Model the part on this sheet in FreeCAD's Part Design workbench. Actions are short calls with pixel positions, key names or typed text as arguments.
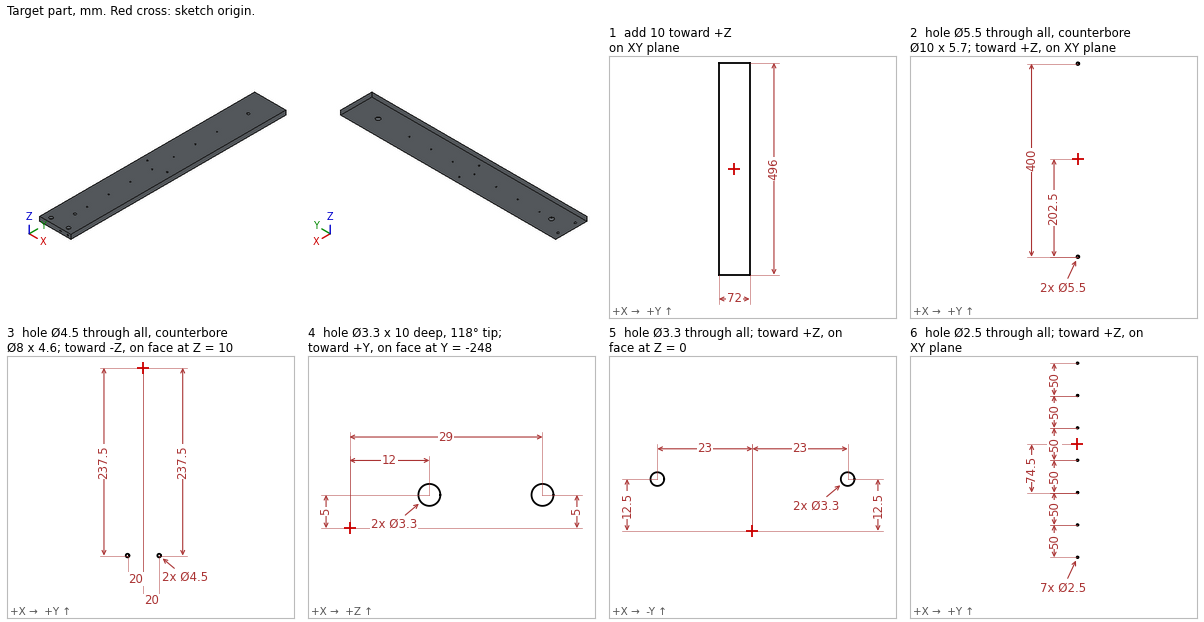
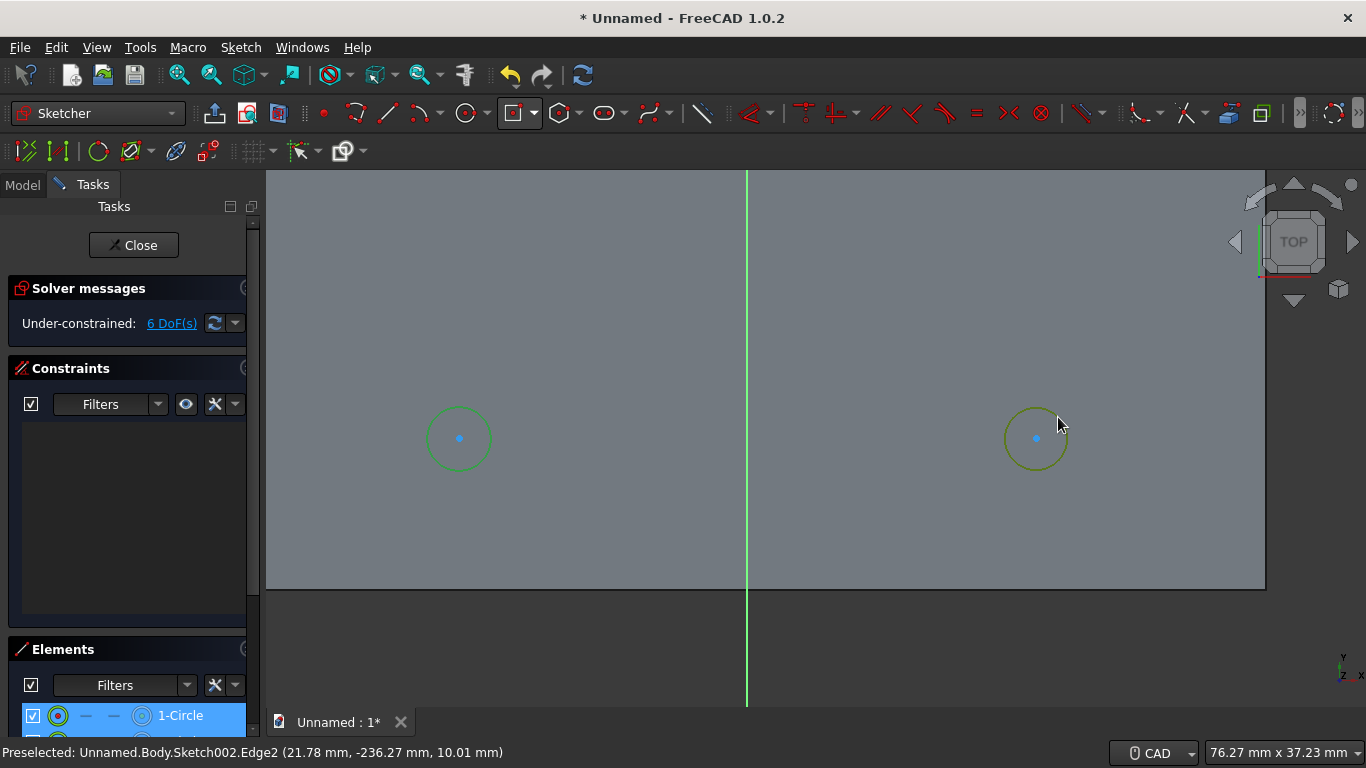
key(e)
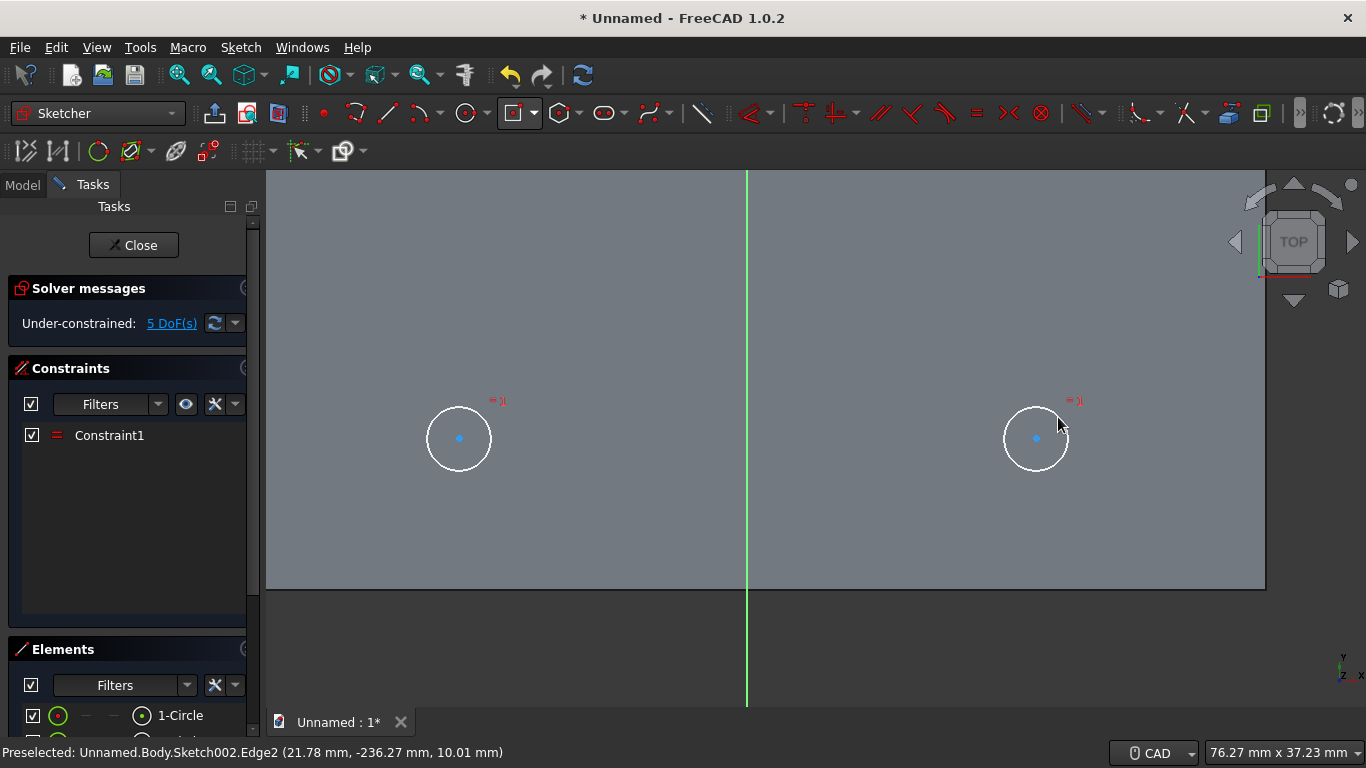
click(750, 114)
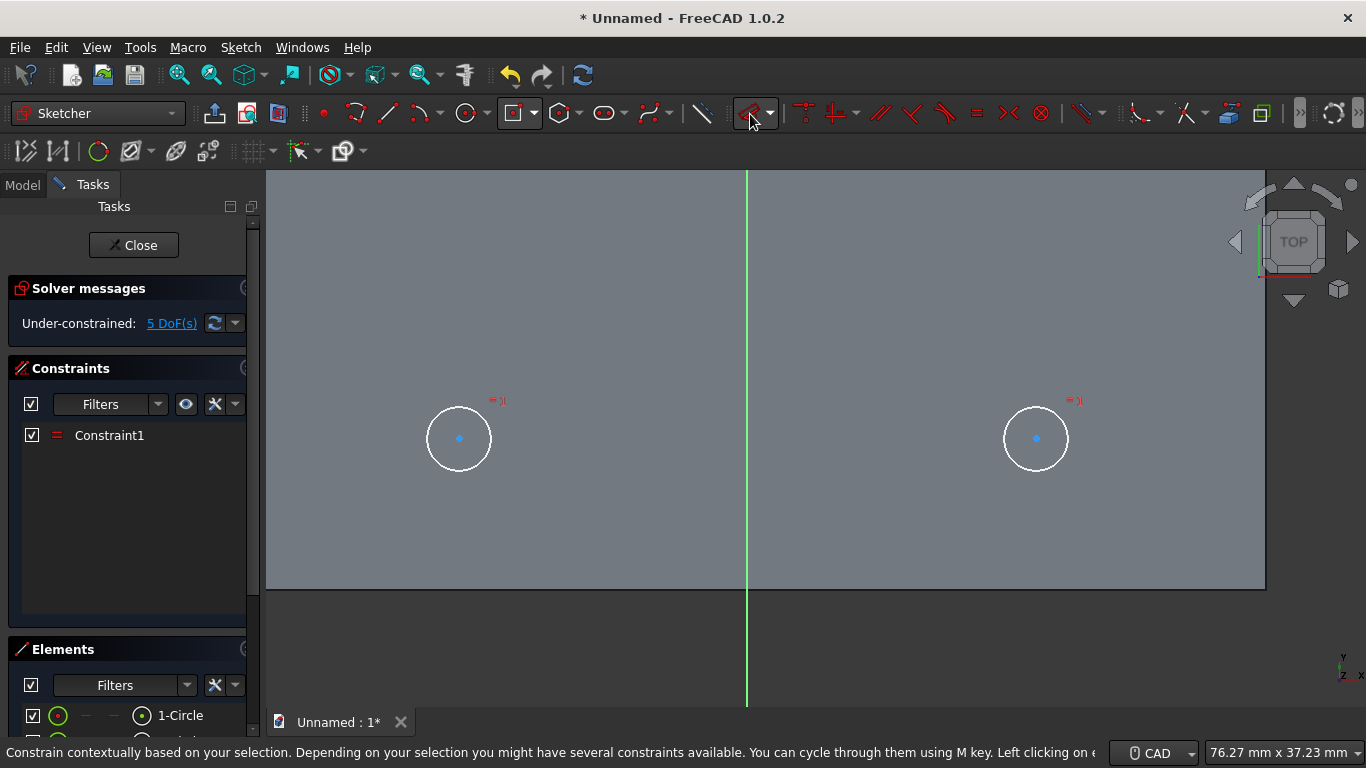
click(481, 416)
click(503, 393)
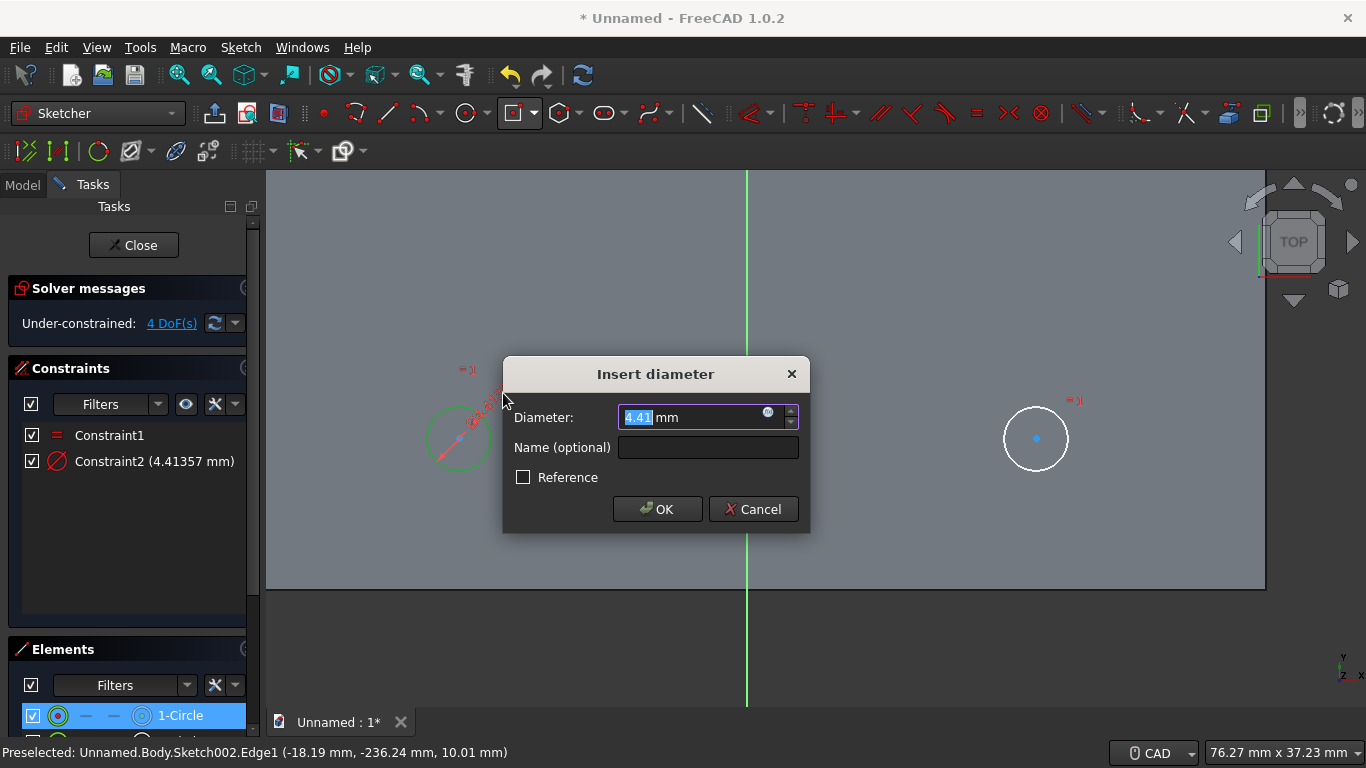
text(4.5)
key(Return)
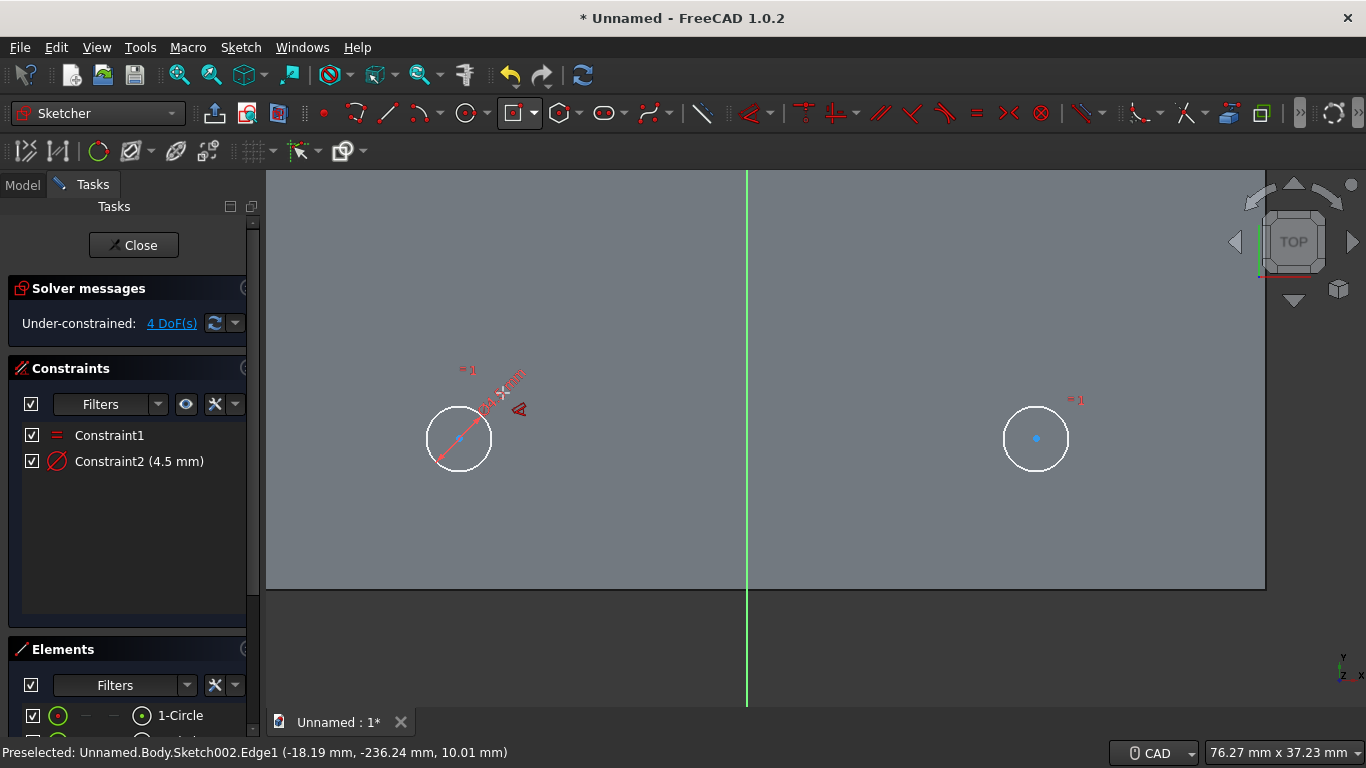
click(459, 439)
click(603, 473)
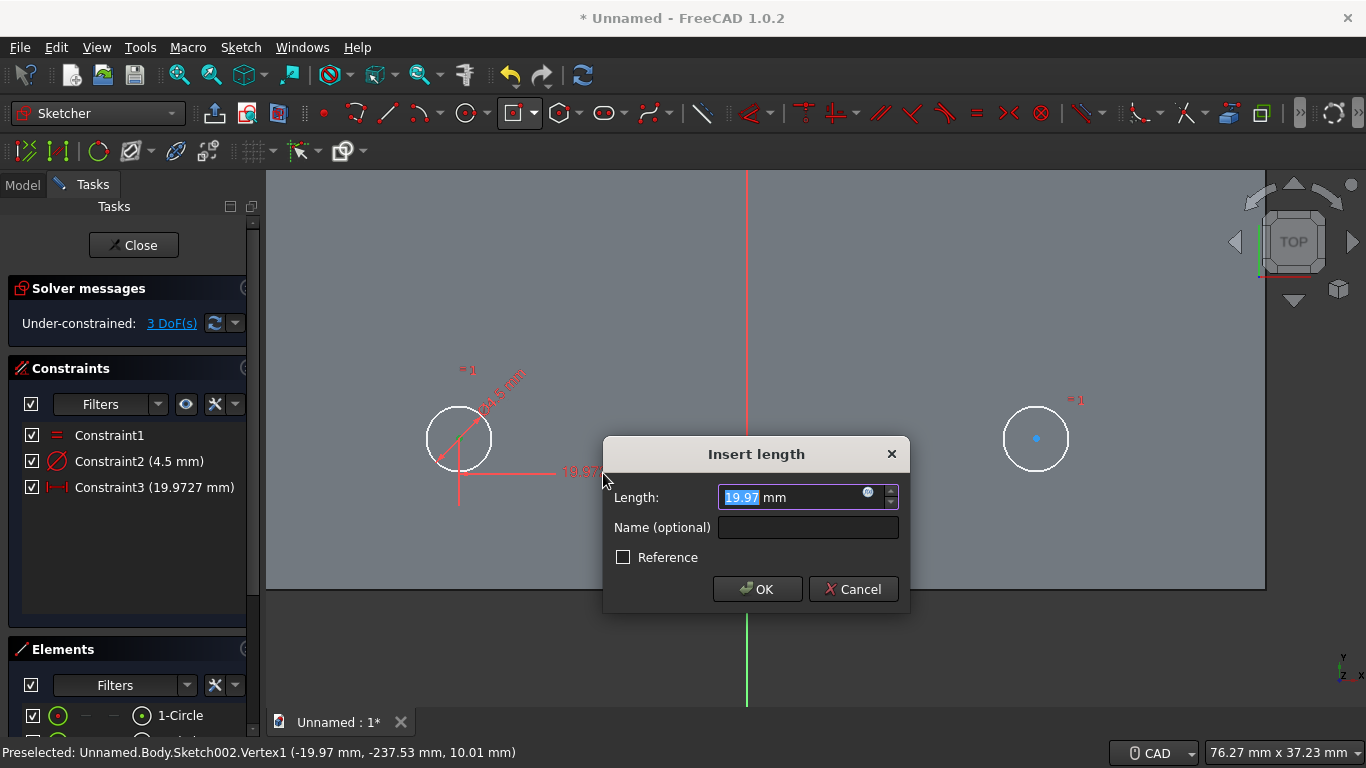
text(20)
key(Return)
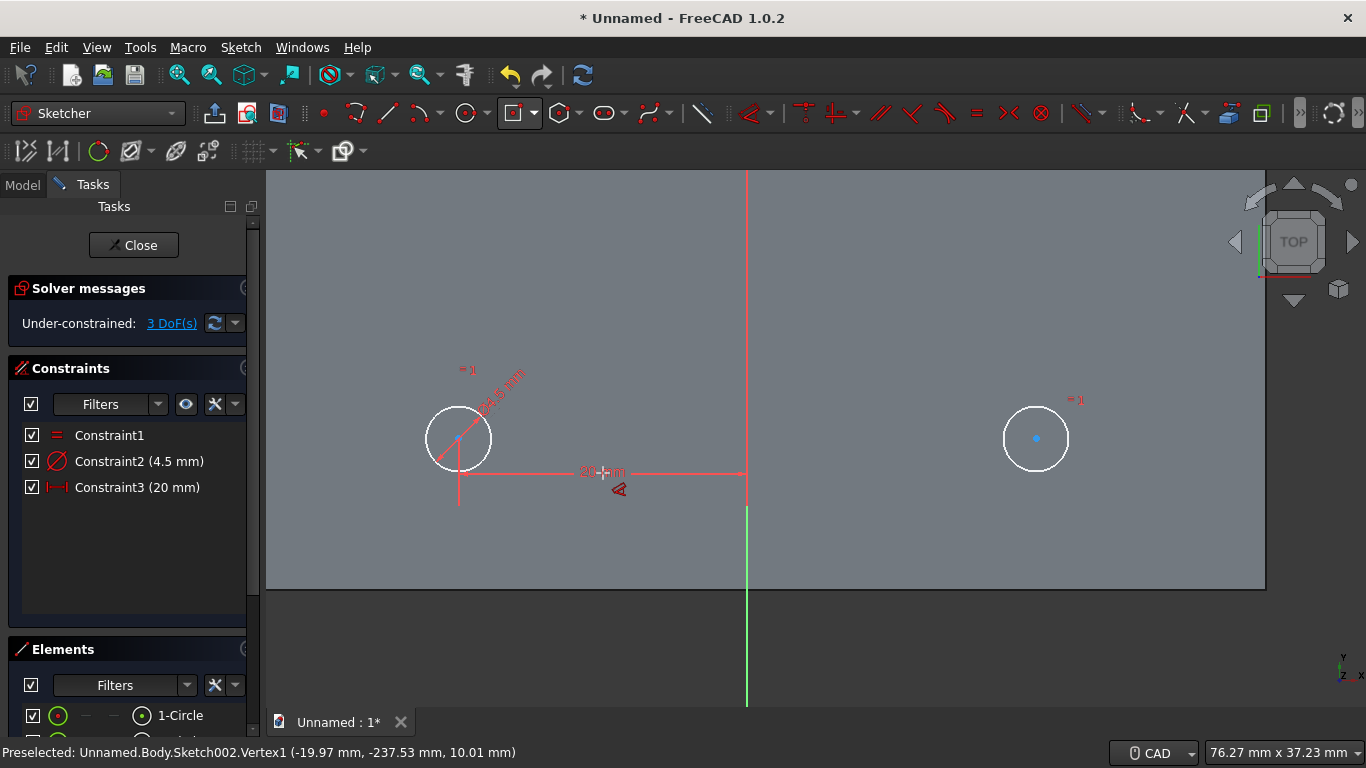
click(1036, 439)
click(892, 473)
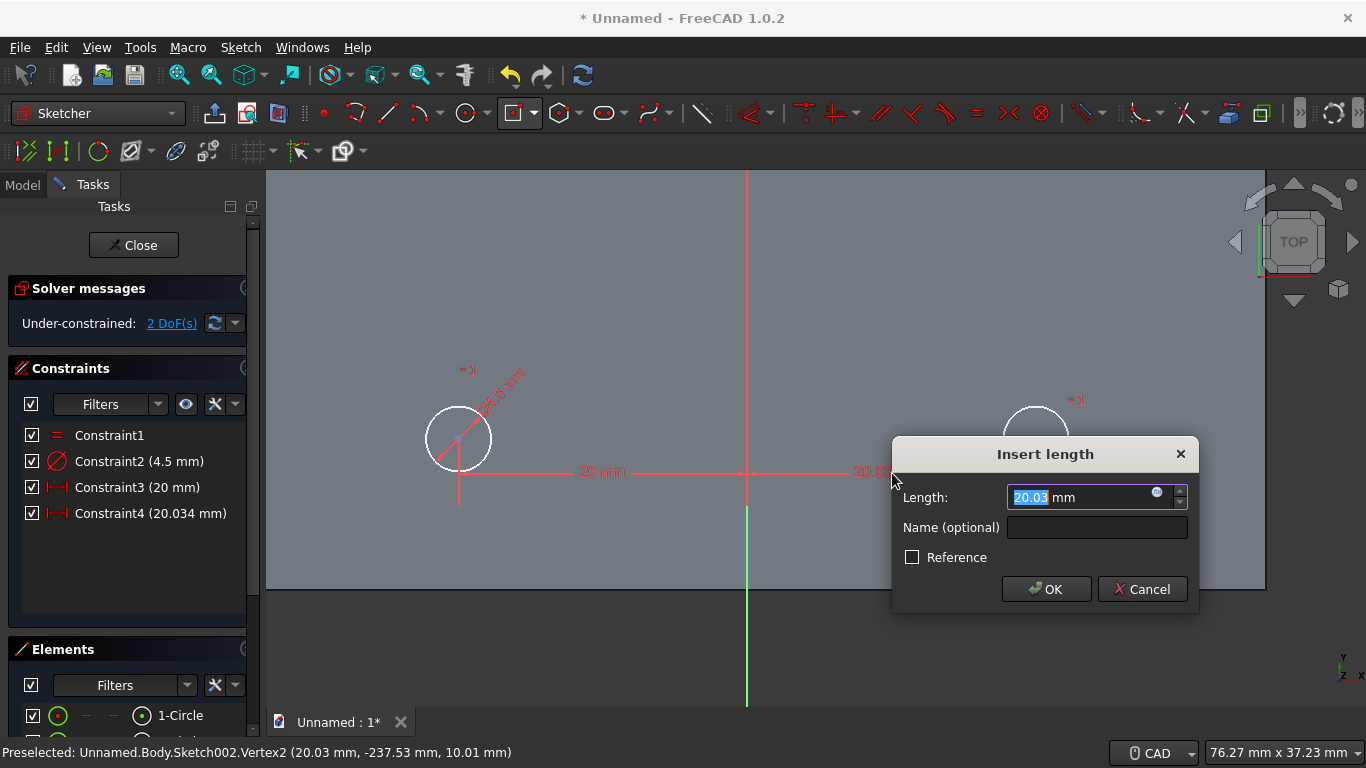
text(20)
key(Return)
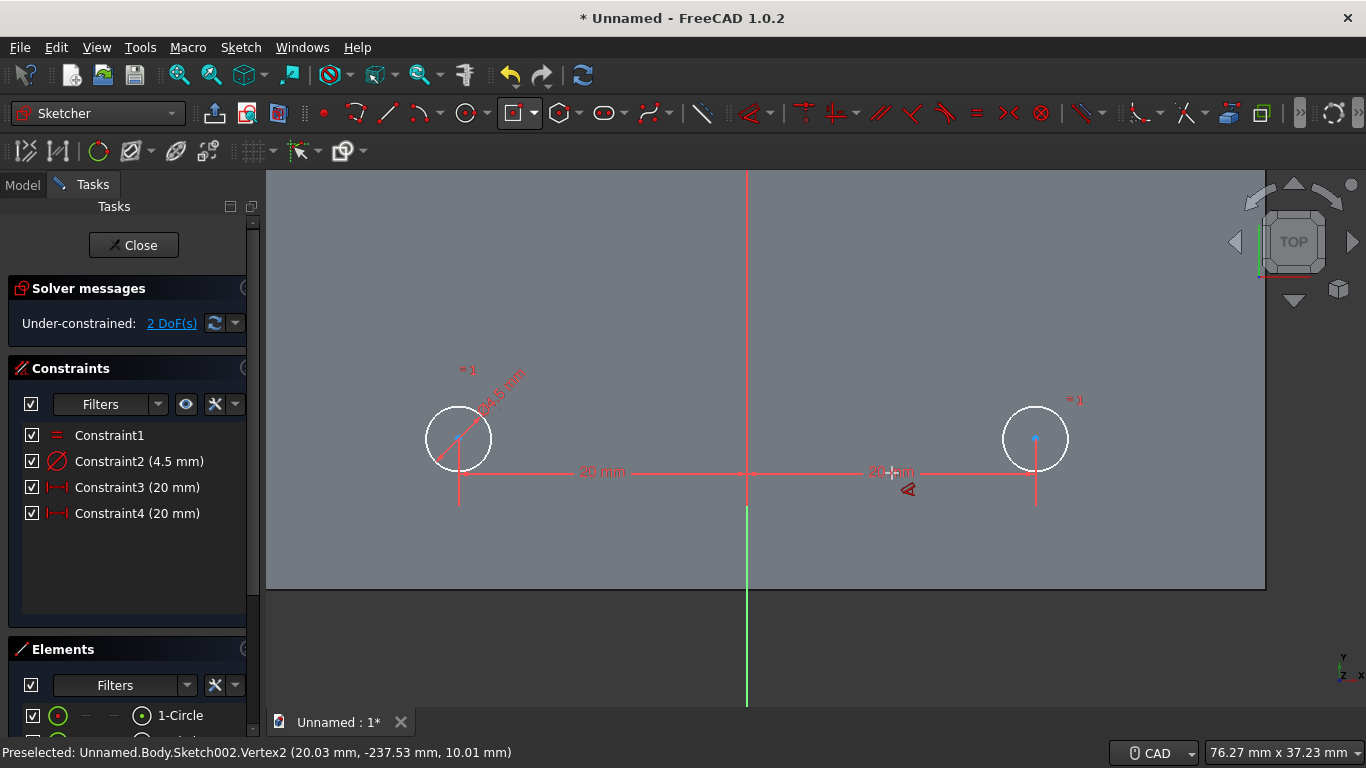
click(459, 439)
click(425, 319)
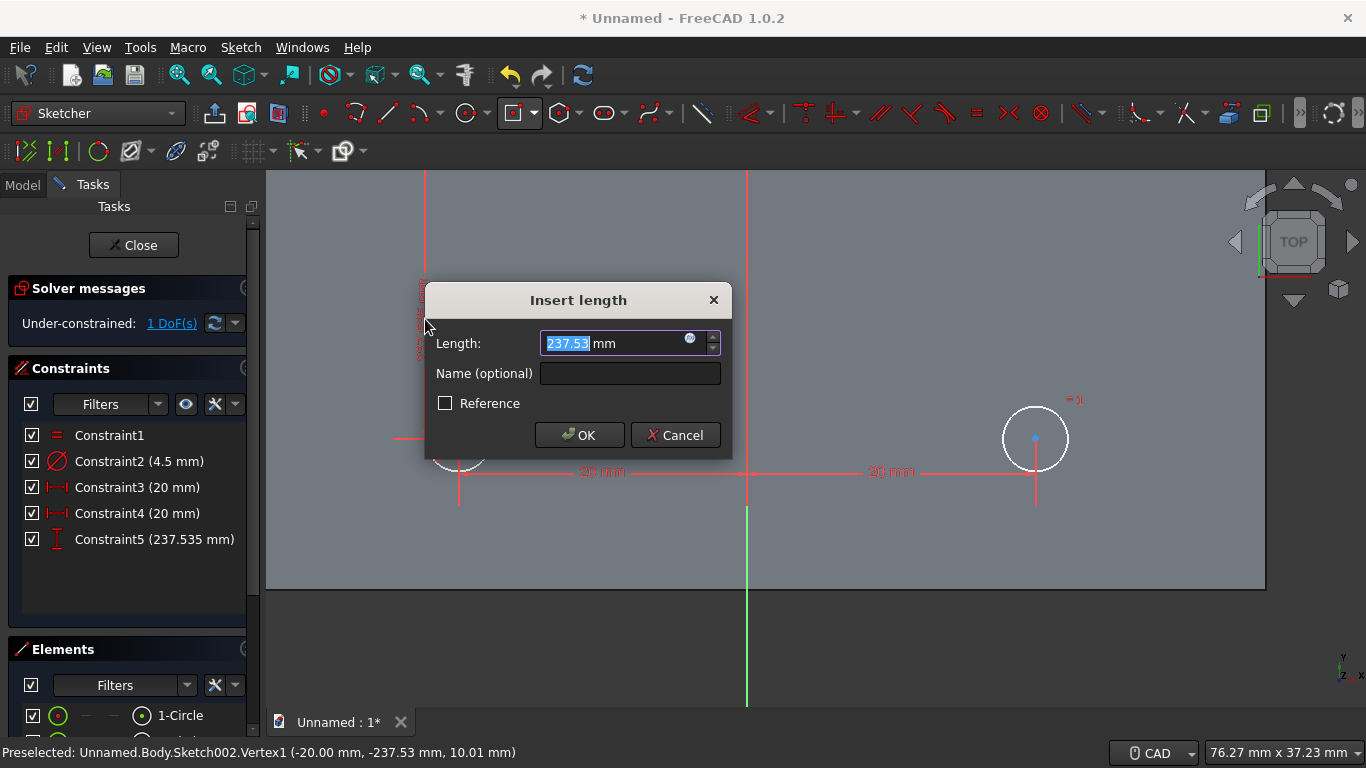
text(237.5)
key(Return)